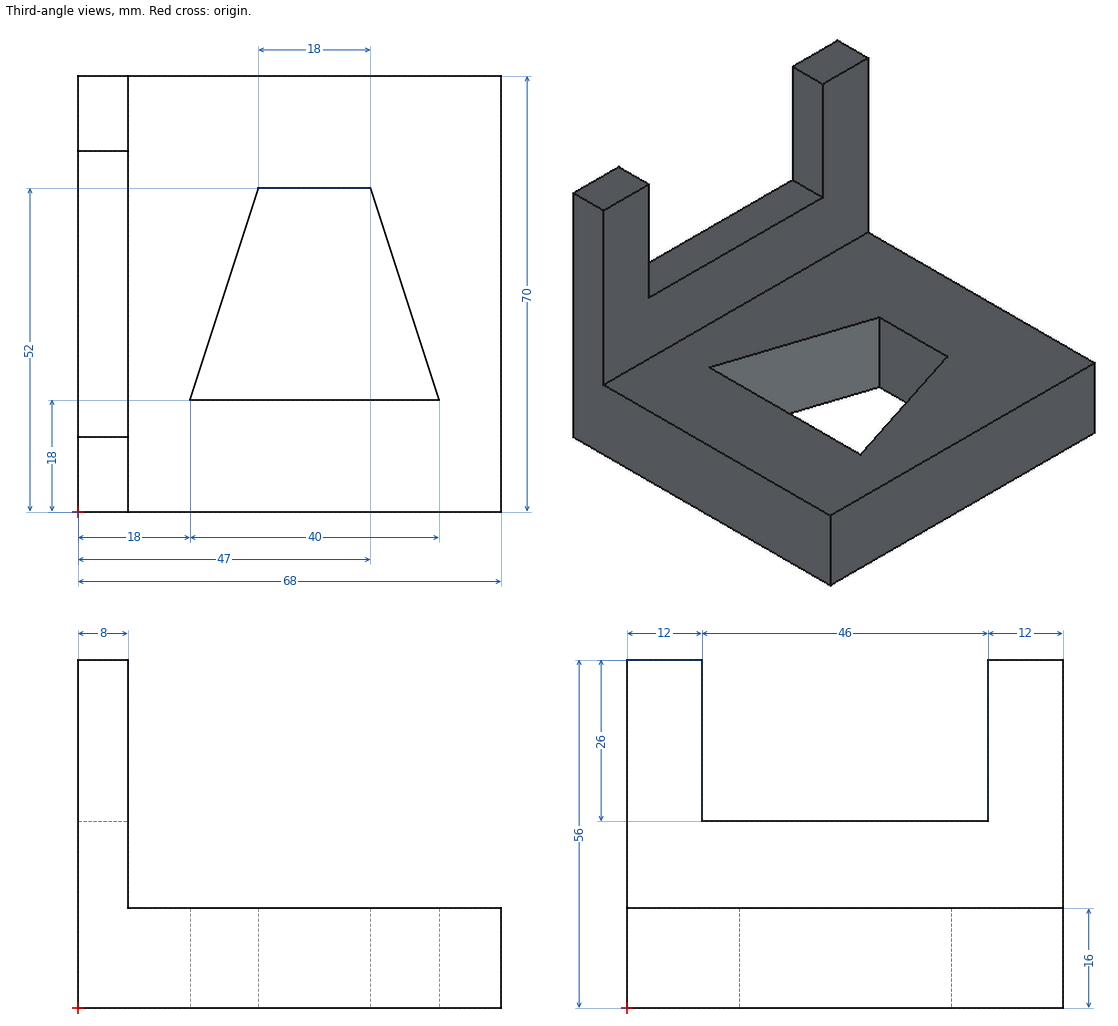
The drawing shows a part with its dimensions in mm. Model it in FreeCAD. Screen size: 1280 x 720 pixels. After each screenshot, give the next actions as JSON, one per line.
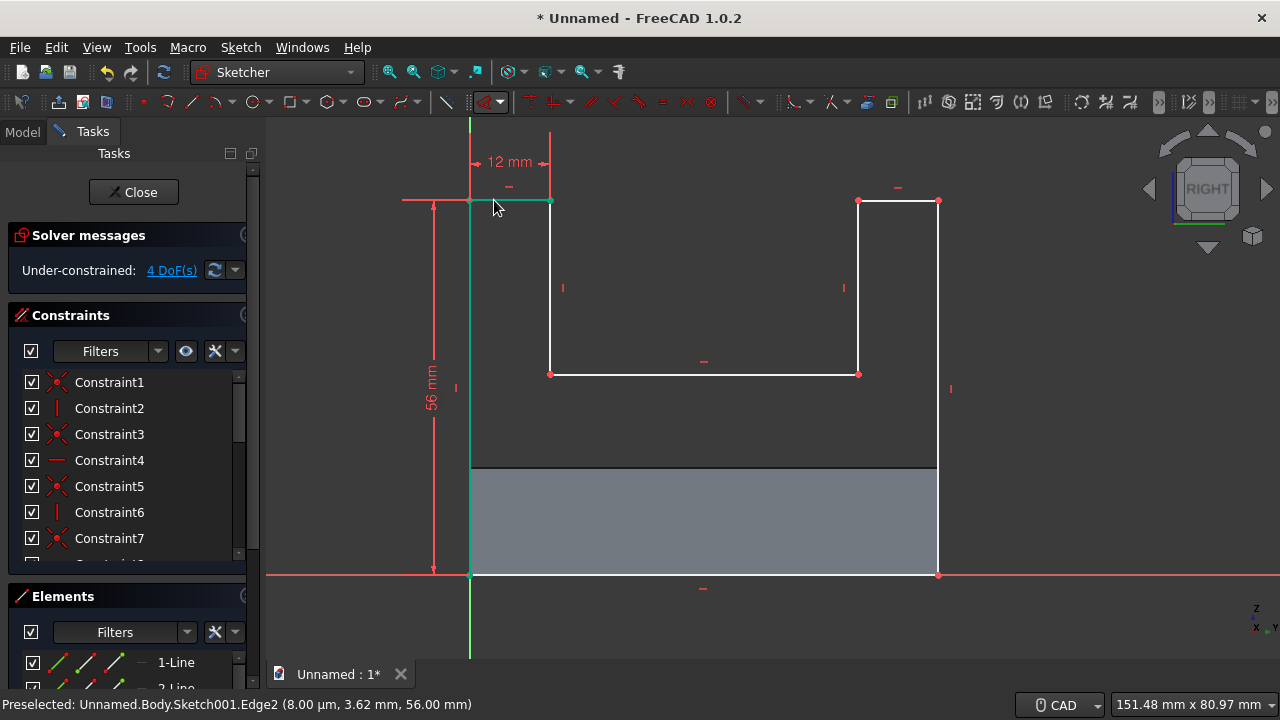
{"action": "left_click", "coordinate": [550, 253]}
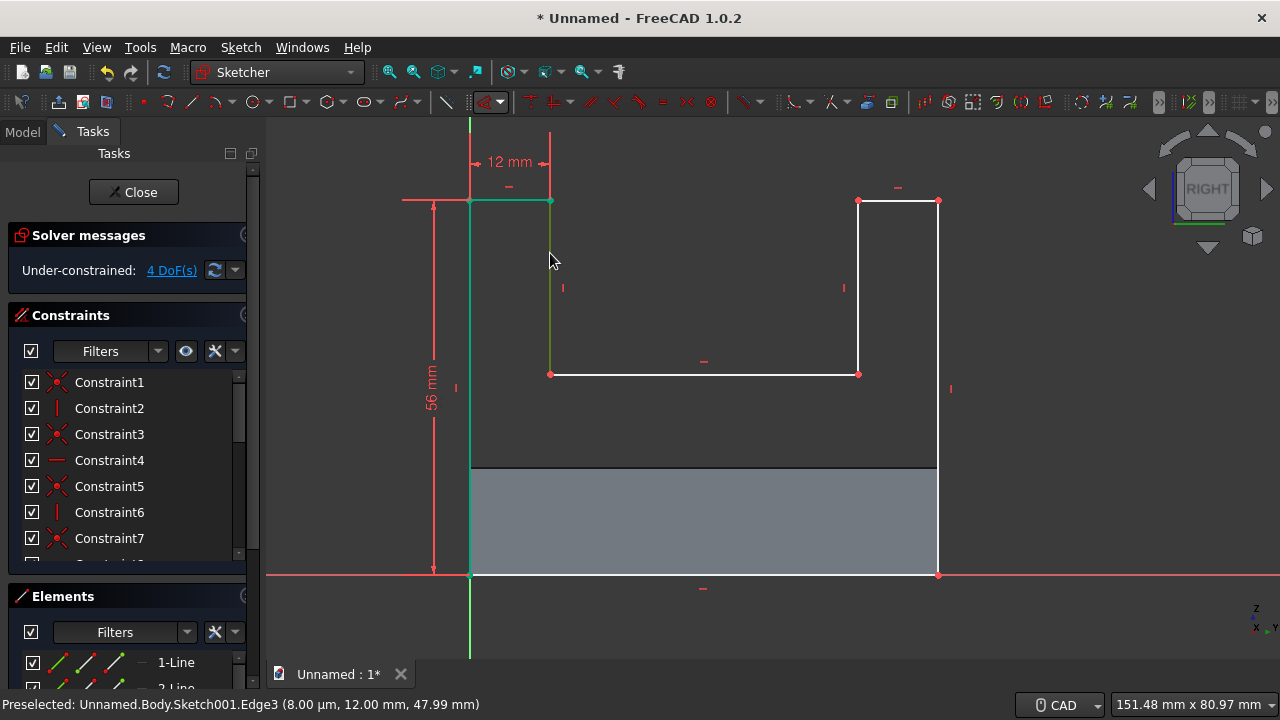
{"action": "key", "text": "i"}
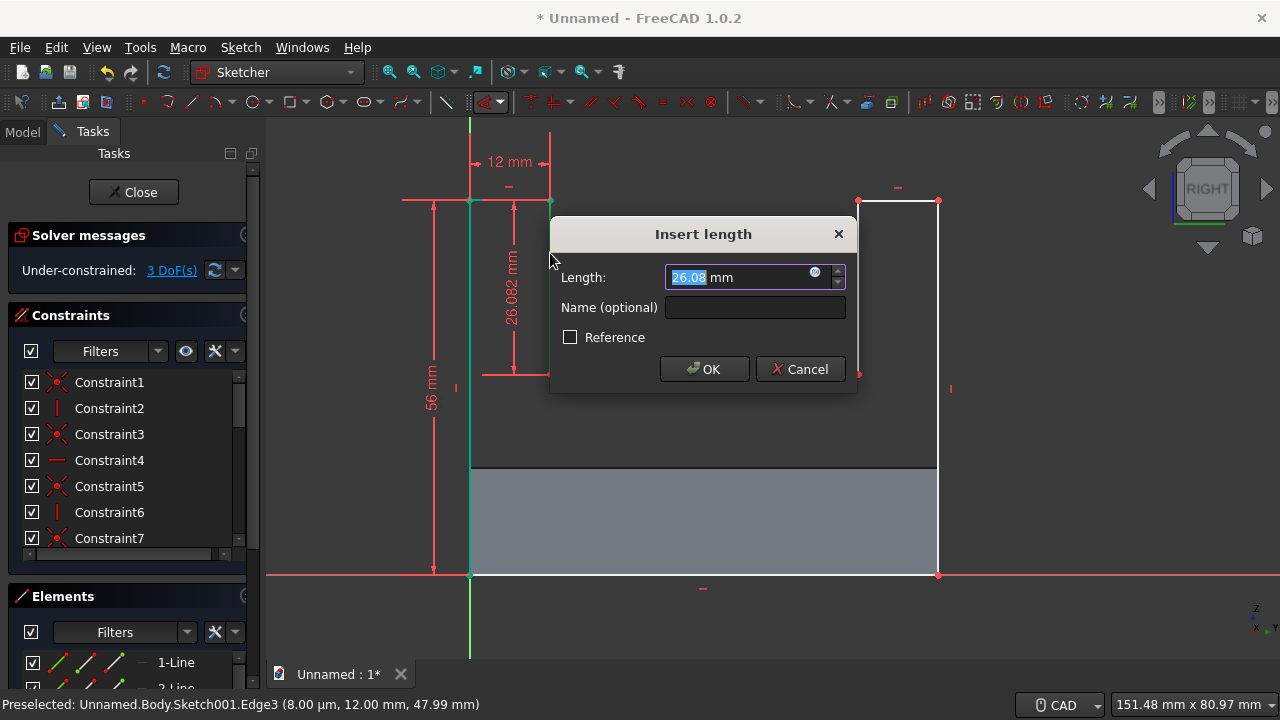
{"action": "type", "text": "26"}
{"action": "key", "text": "Return"}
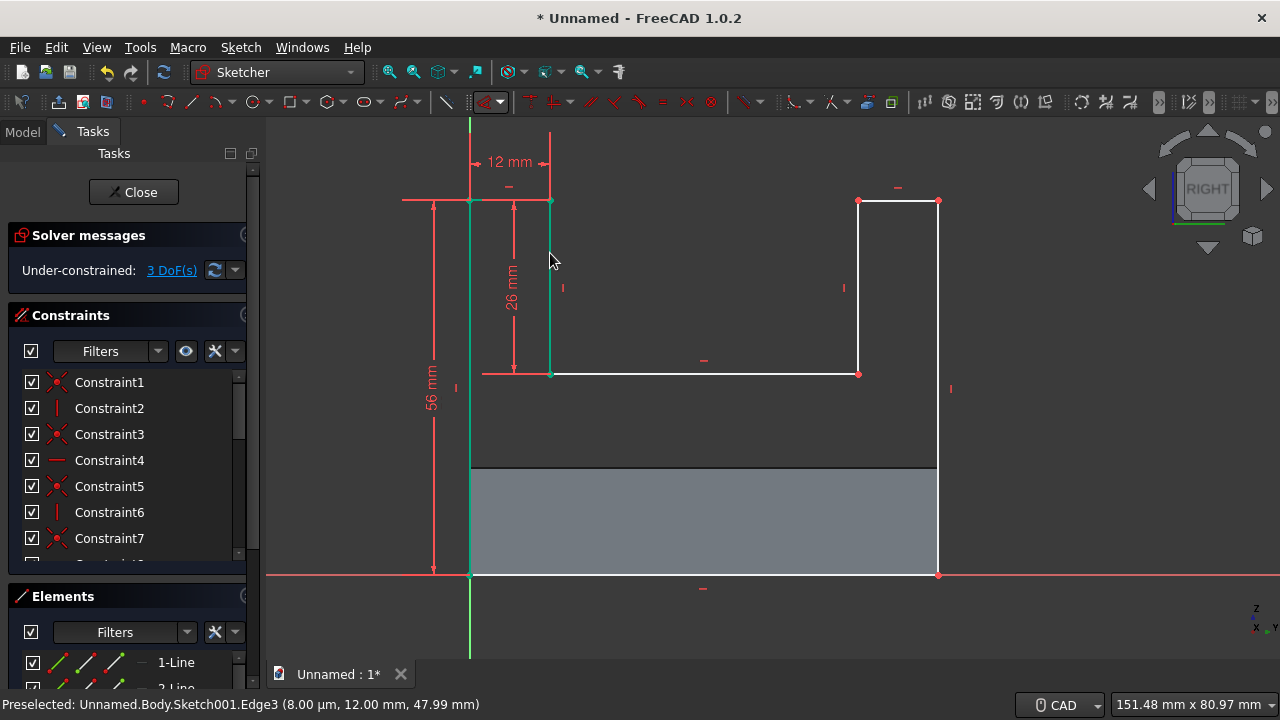
{"action": "left_click", "coordinate": [642, 374]}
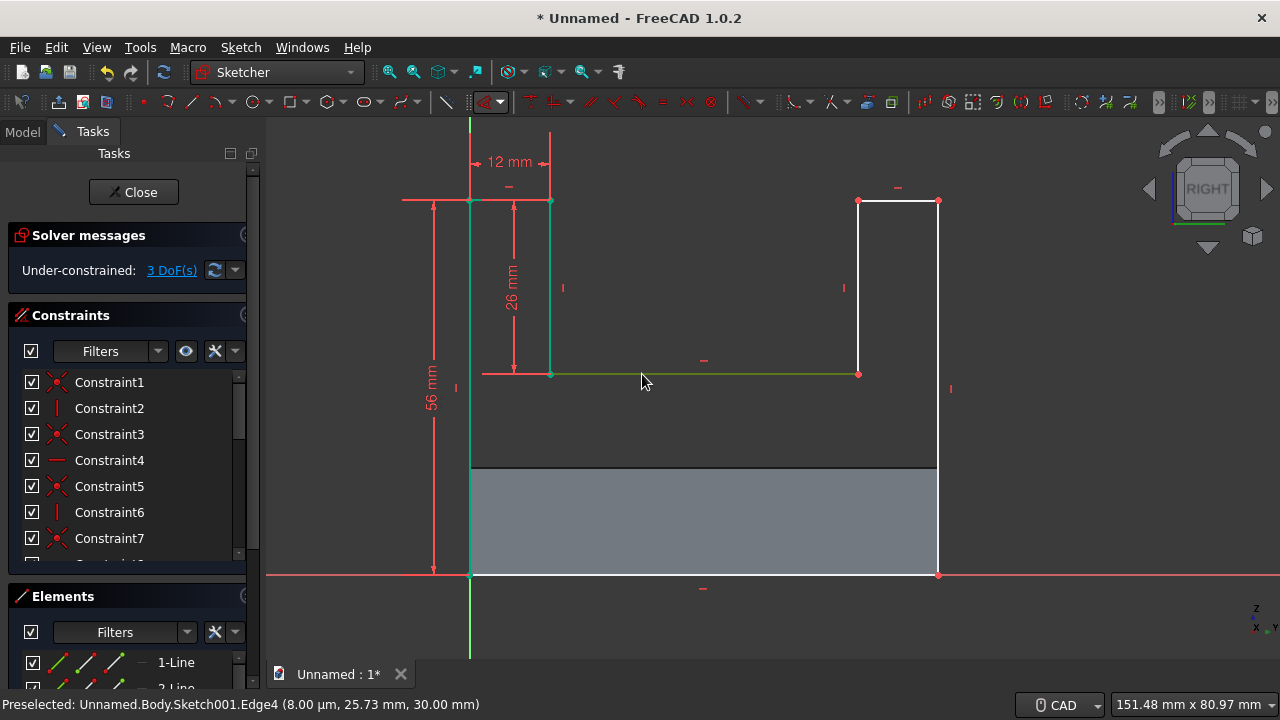
{"action": "key", "text": "l"}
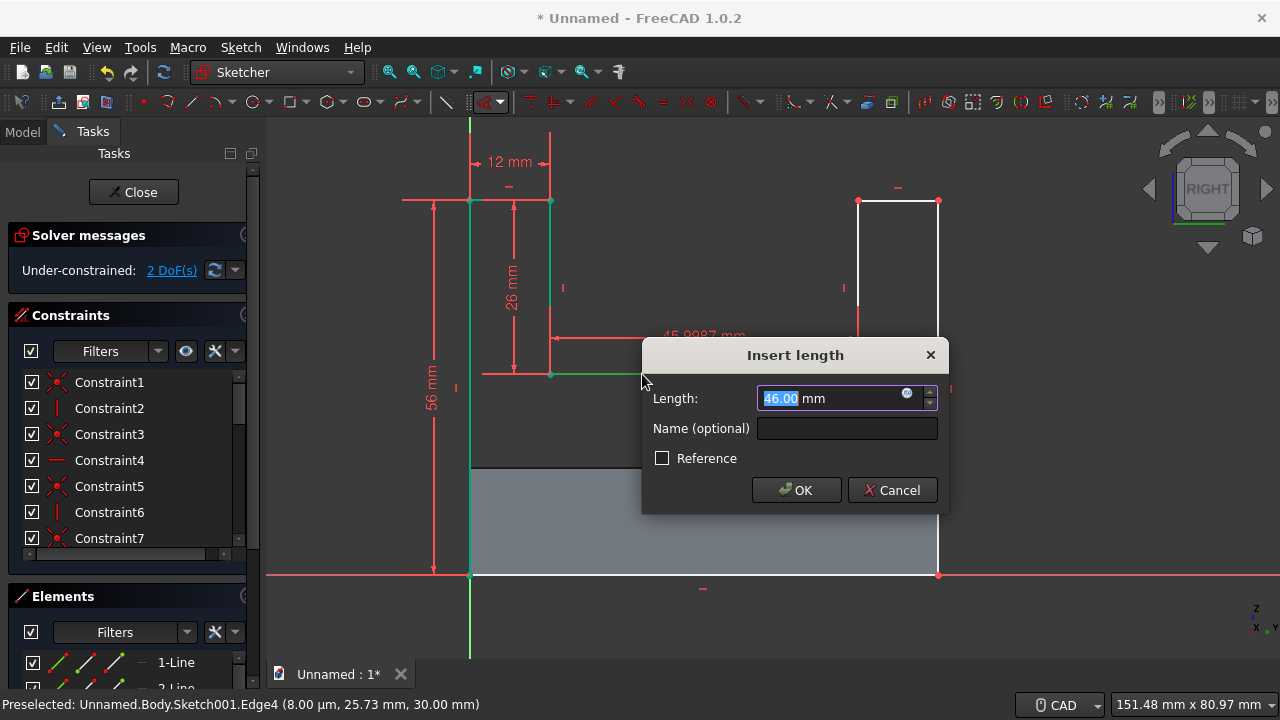
{"action": "type", "text": "46"}
{"action": "key", "text": "Return"}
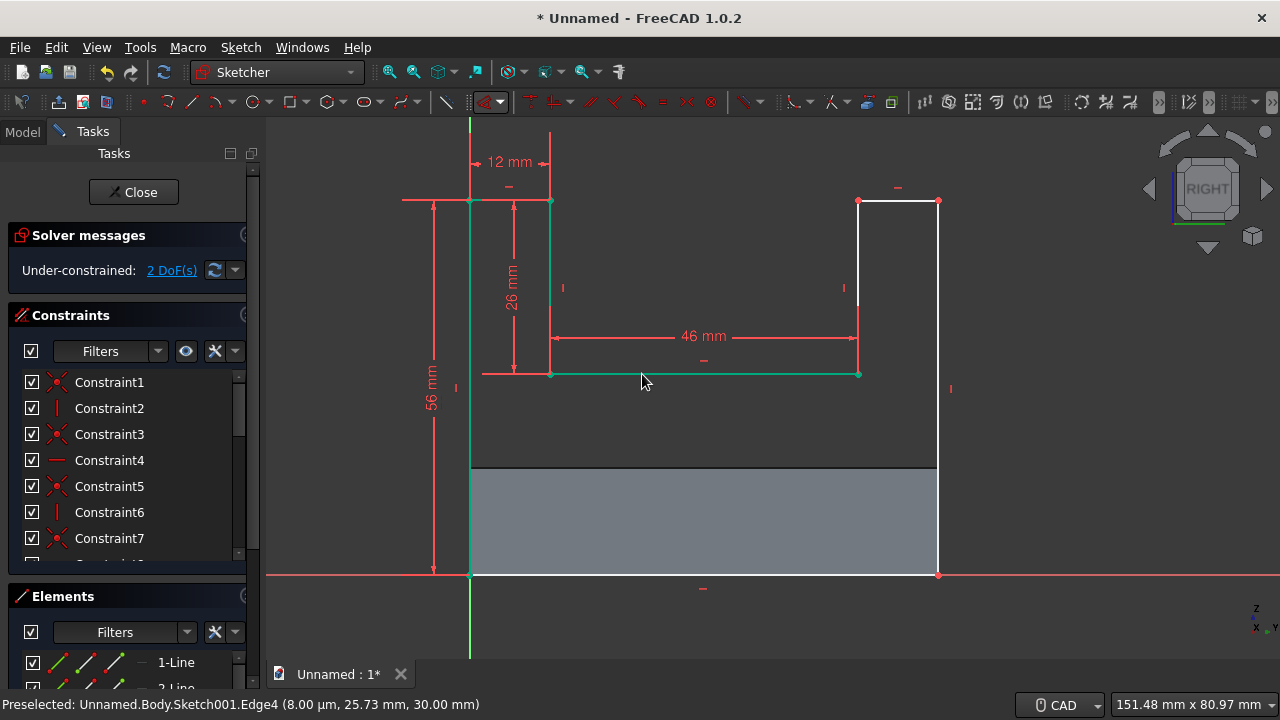
{"action": "left_click", "coordinate": [858, 322]}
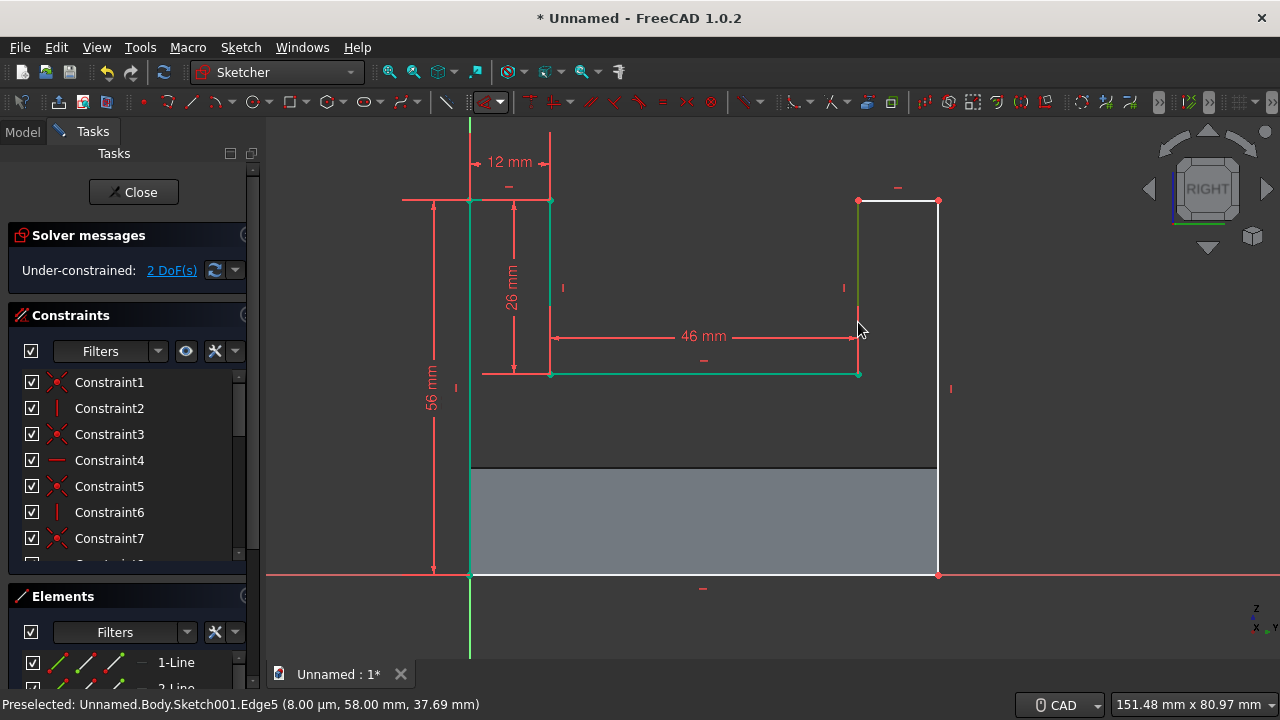
{"action": "key", "text": "i"}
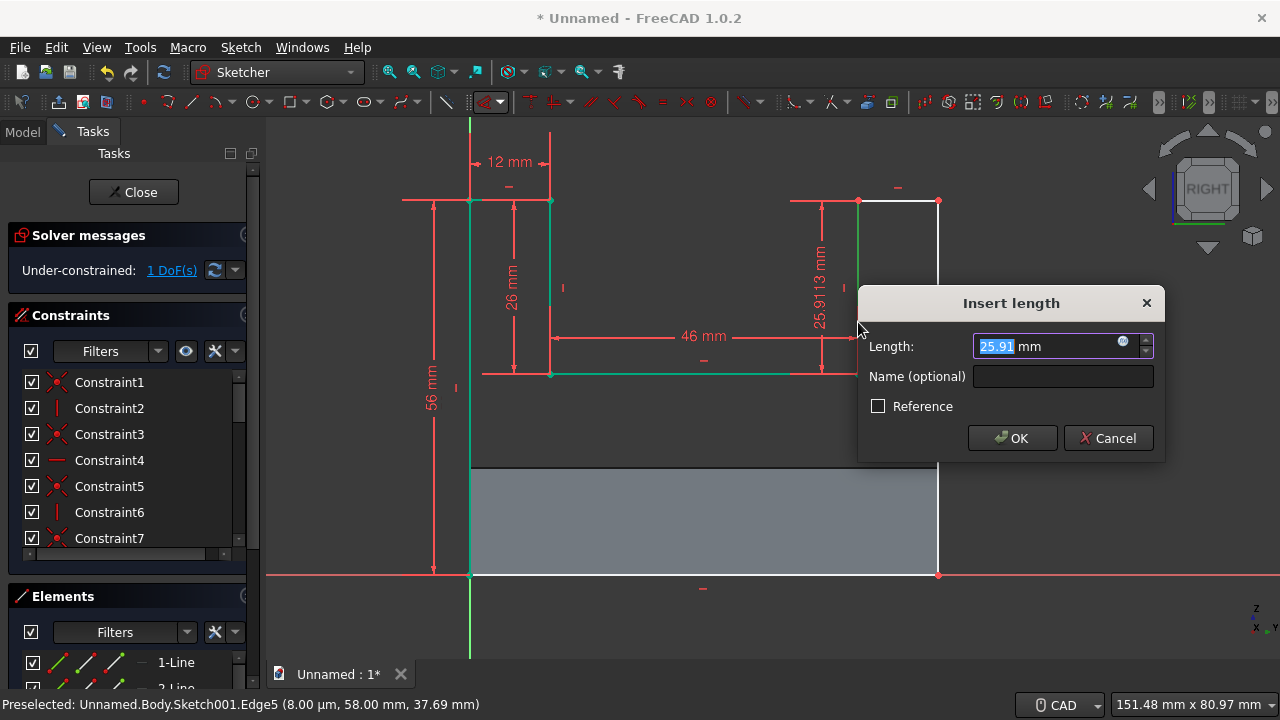
{"action": "type", "text": "26"}
{"action": "key", "text": "Return"}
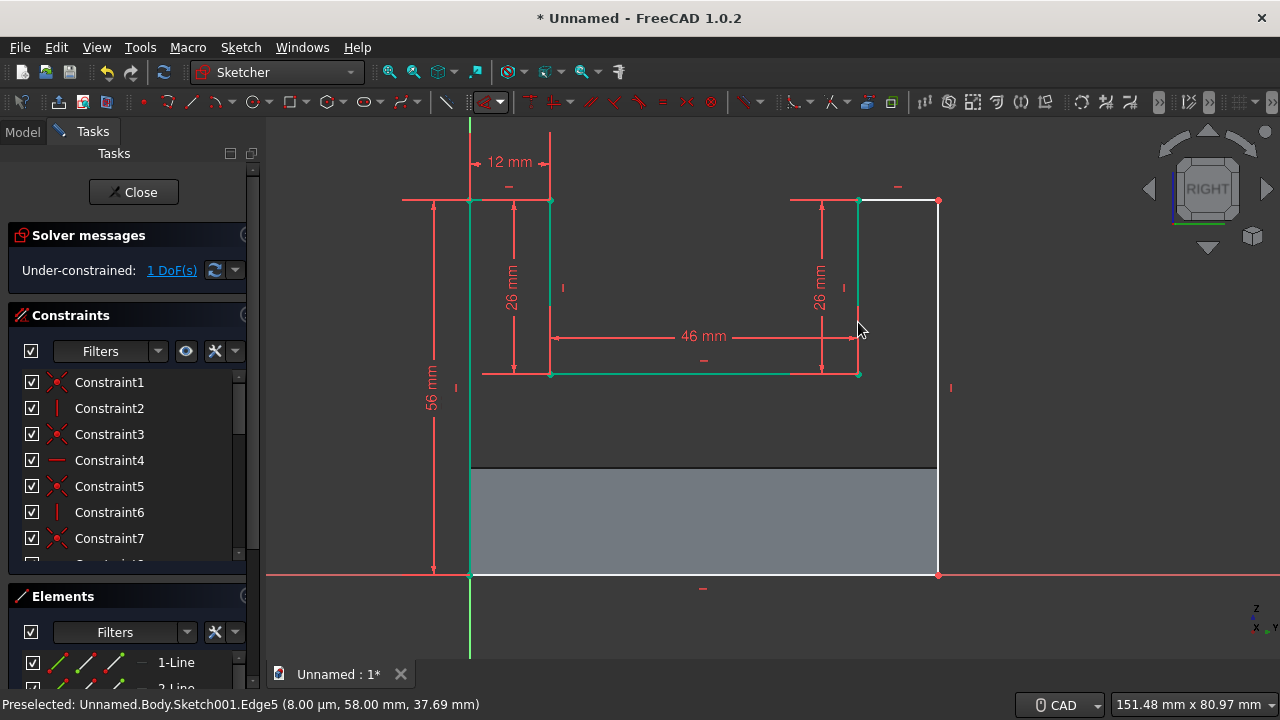
{"action": "left_click", "coordinate": [882, 200]}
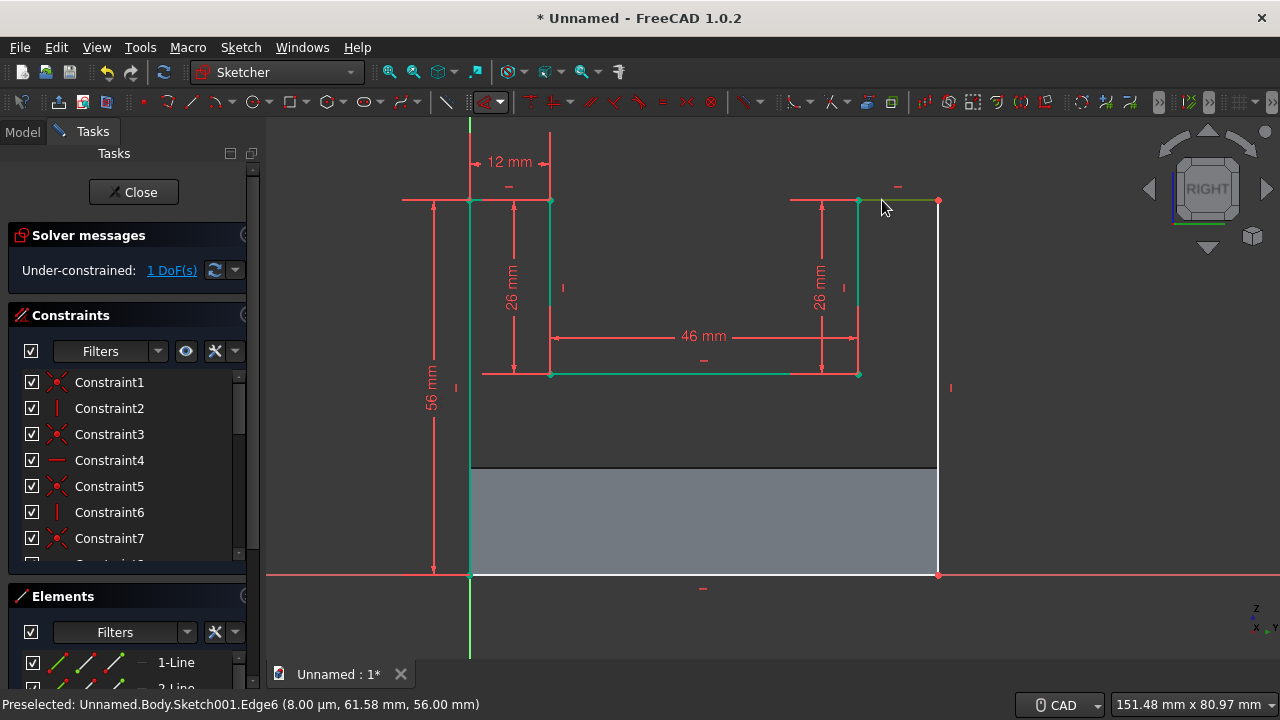
{"action": "left_click", "coordinate": [502, 102]}